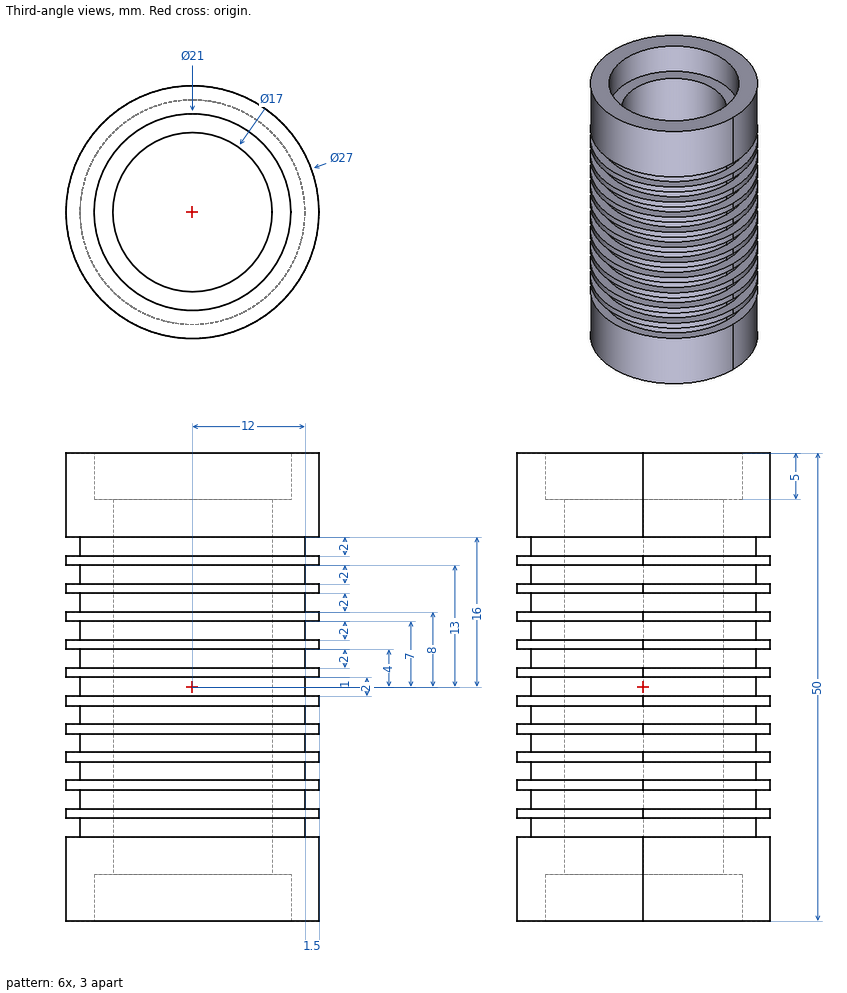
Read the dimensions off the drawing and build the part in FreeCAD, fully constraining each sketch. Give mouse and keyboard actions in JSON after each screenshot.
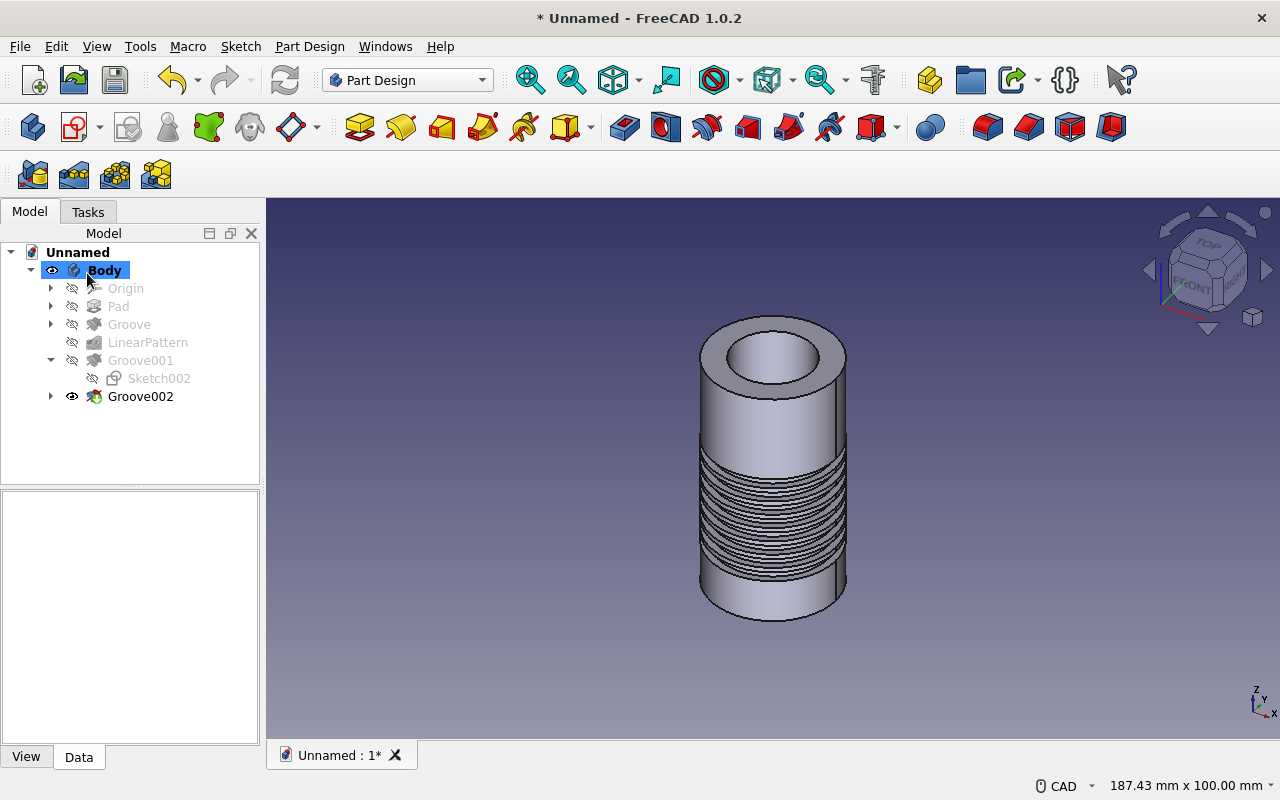
{"action": "left_click", "coordinate": [74, 128]}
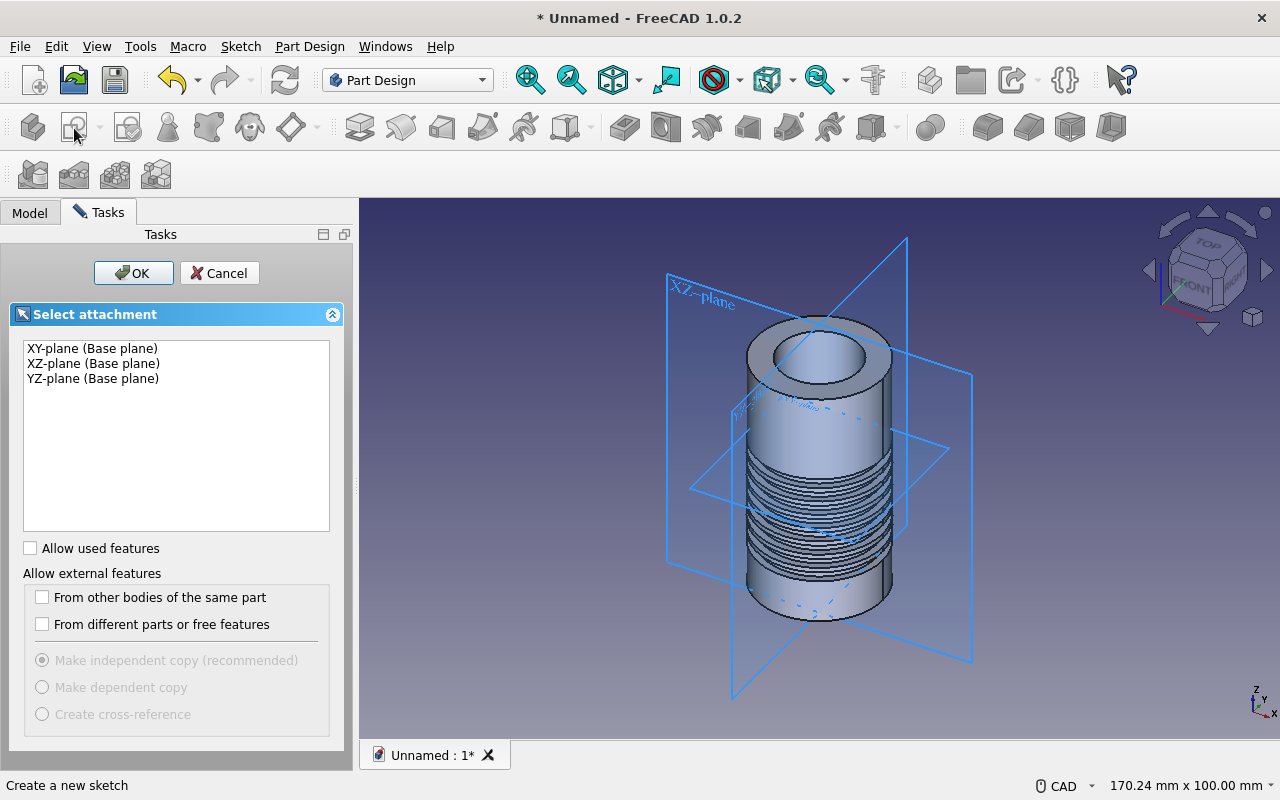
{"action": "left_click", "coordinate": [84, 364]}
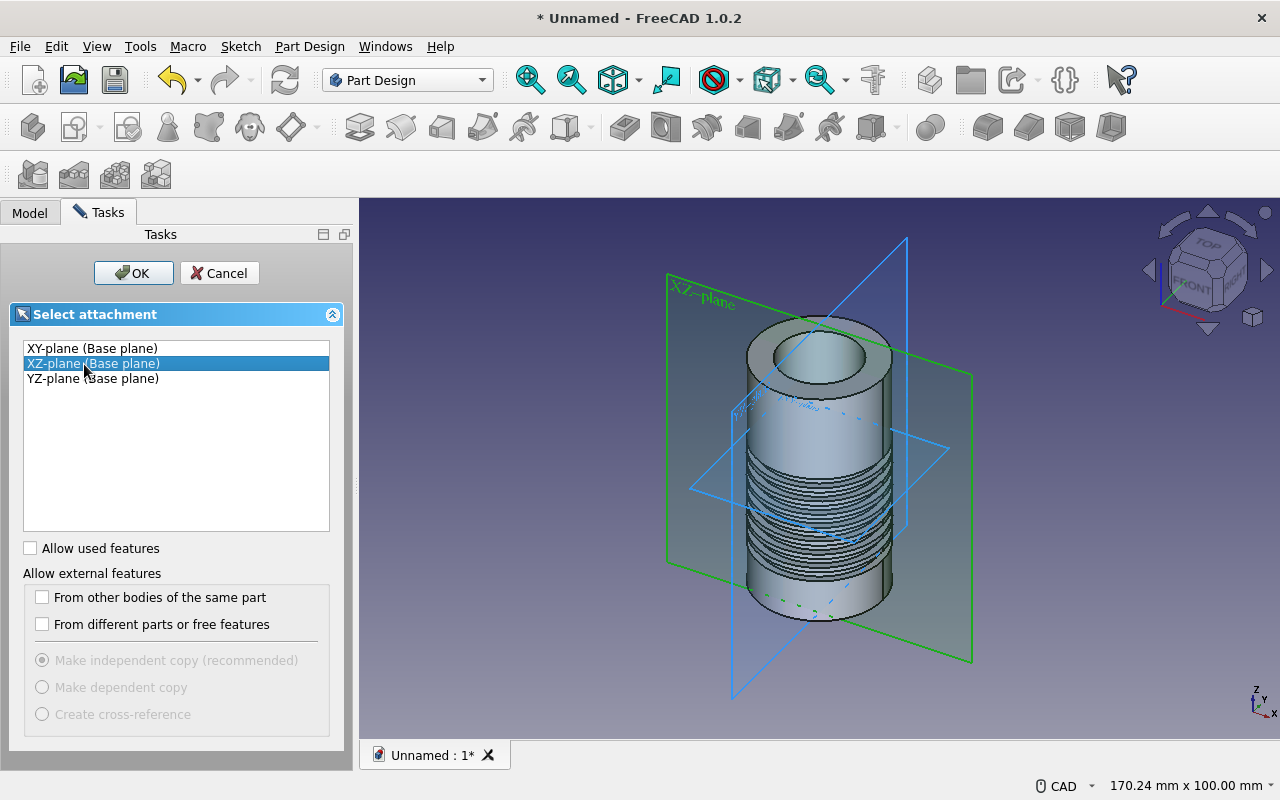
{"action": "left_click", "coordinate": [134, 273]}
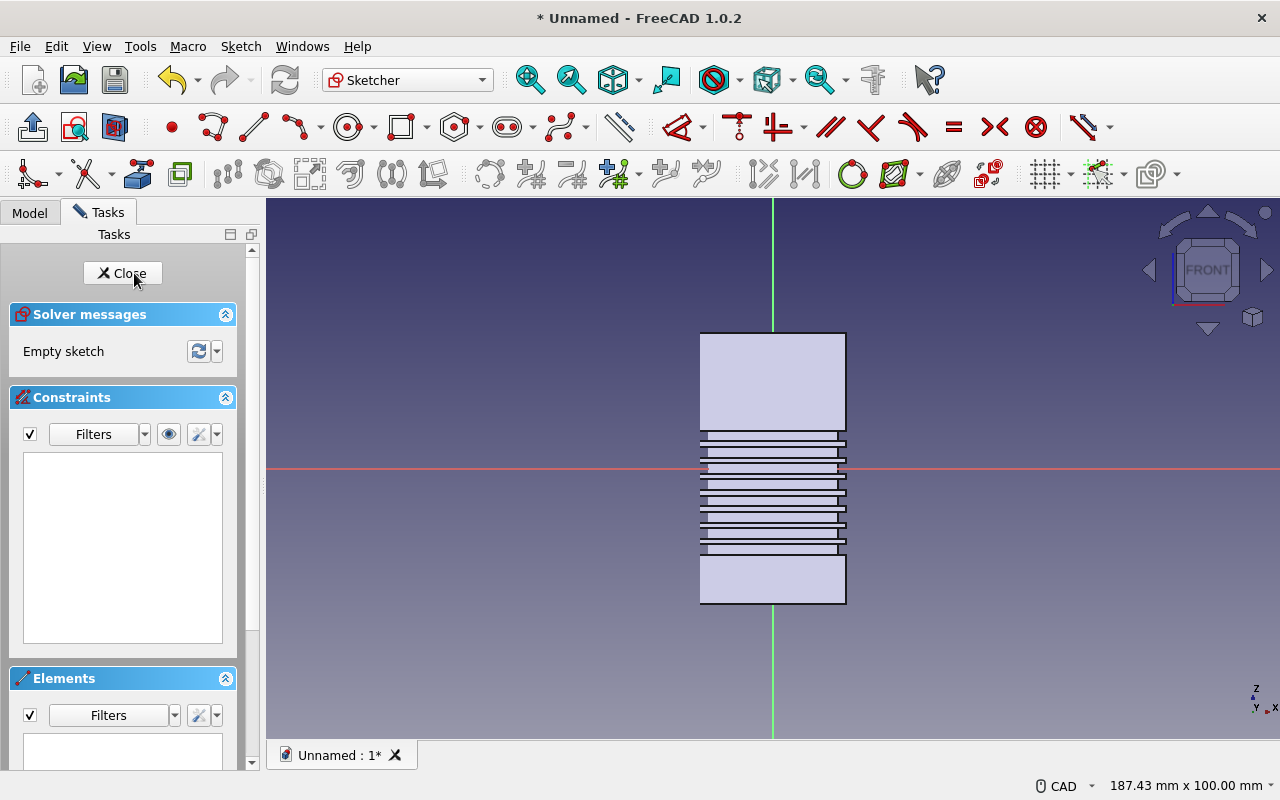
{"action": "key", "text": "q s"}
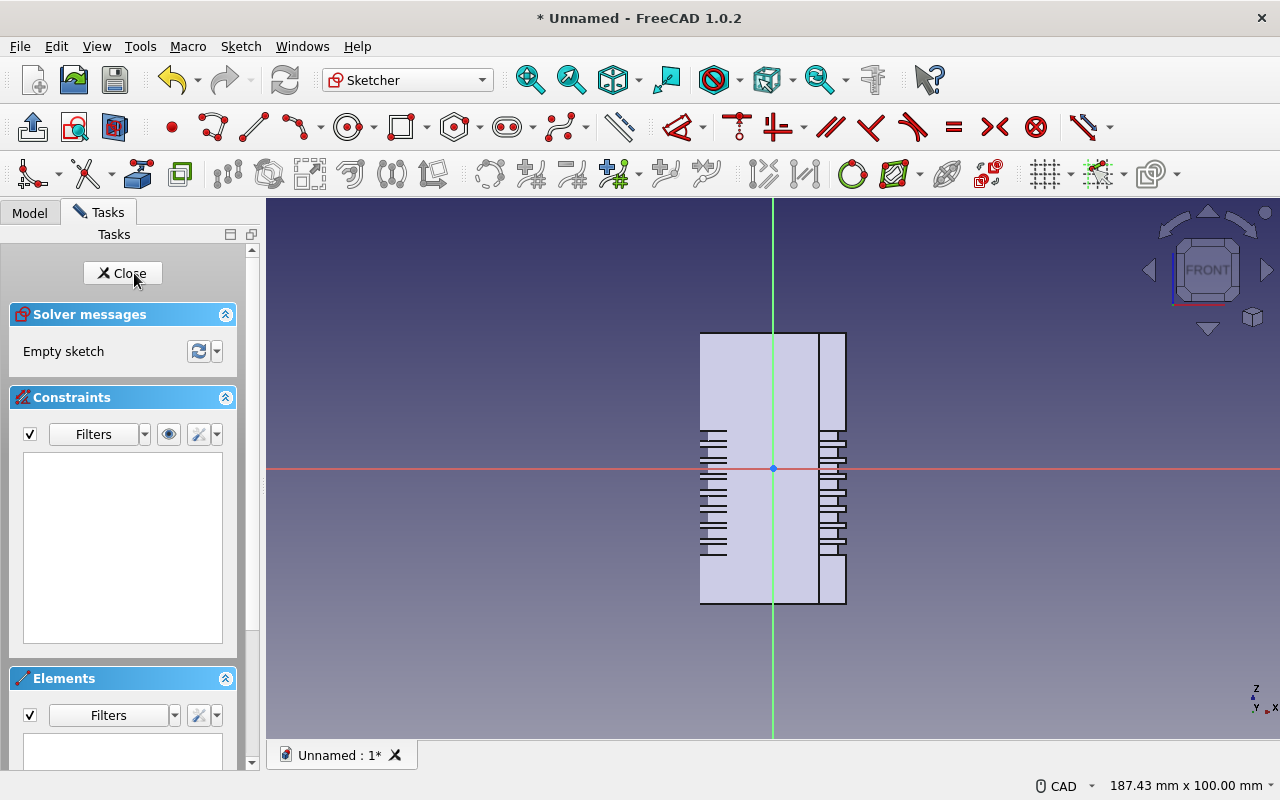
{"action": "scroll", "coordinate": [849, 417], "scroll_direction": "up", "scroll_amount": 15}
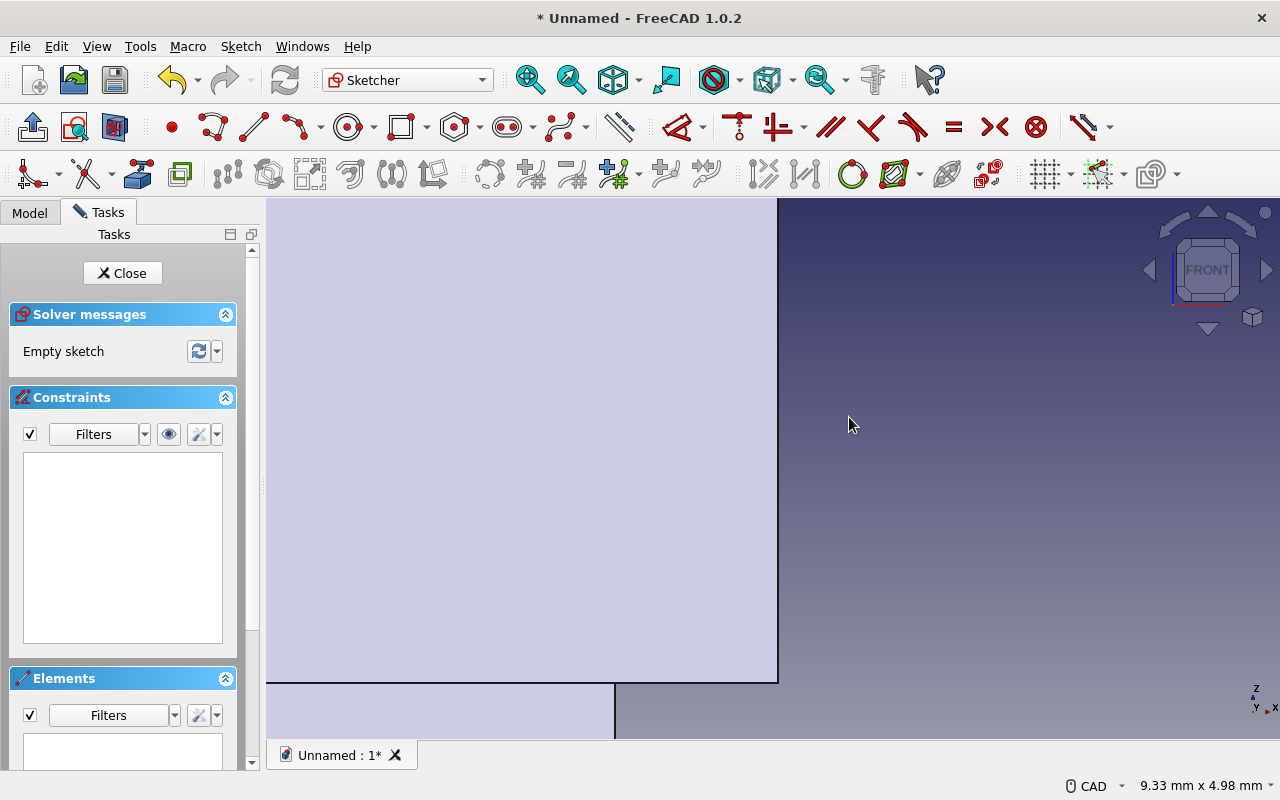
{"action": "scroll", "coordinate": [682, 460], "scroll_direction": "up", "scroll_amount": 2}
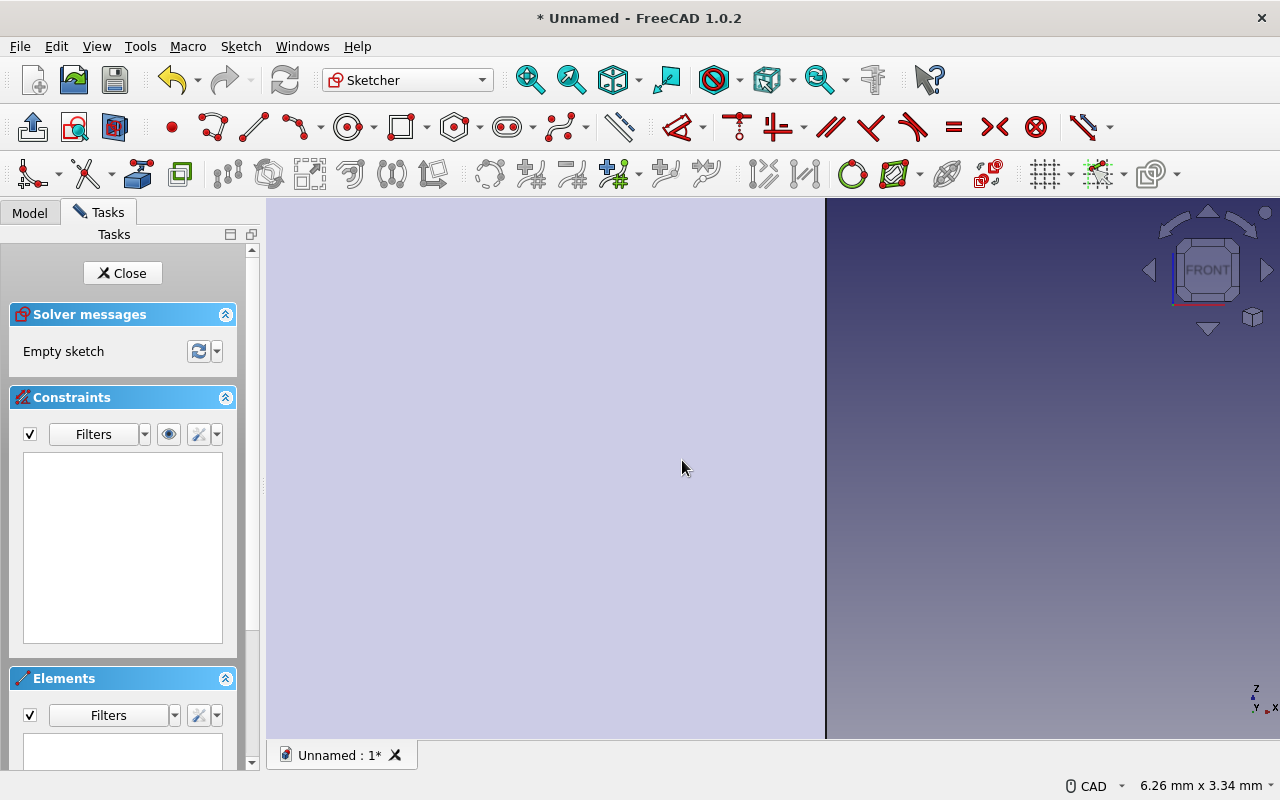
{"action": "left_click", "coordinate": [400, 128]}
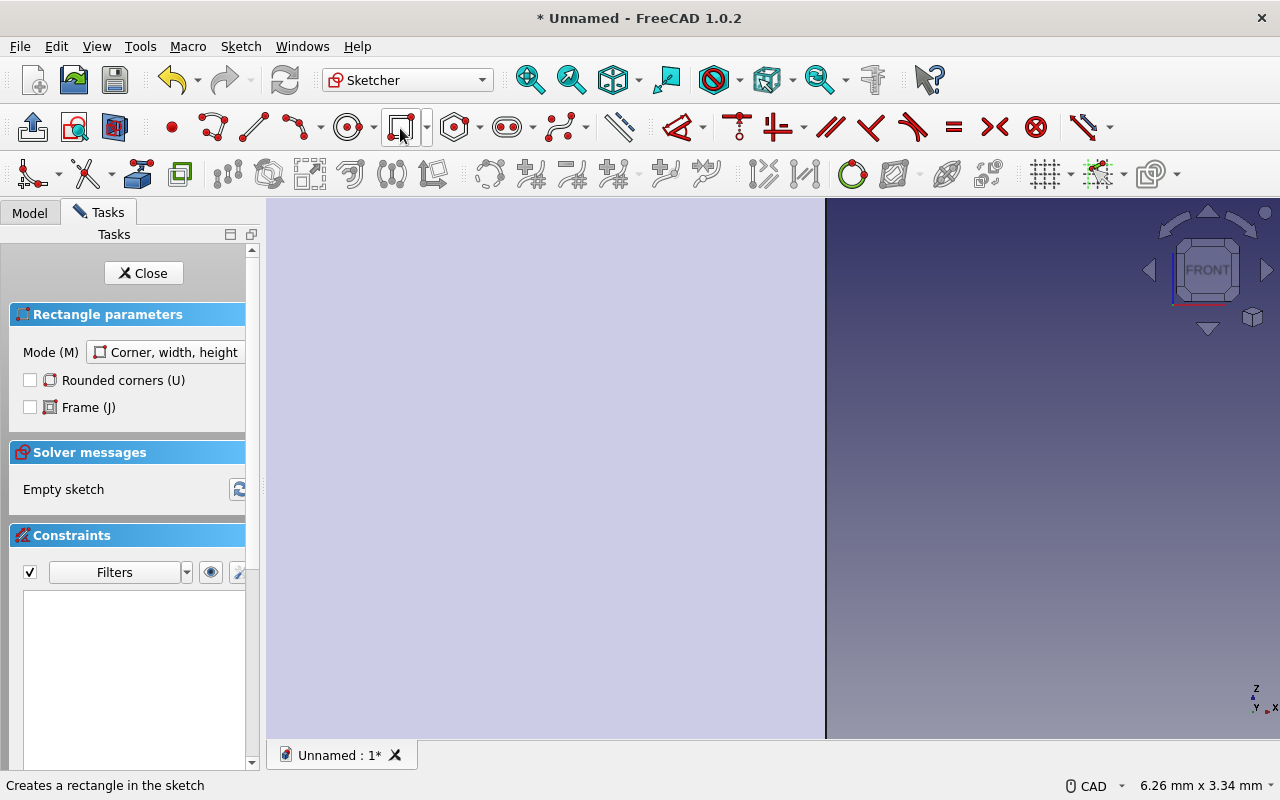
{"action": "left_click", "coordinate": [583, 306]}
{"action": "mouse_move", "coordinate": [826, 630]}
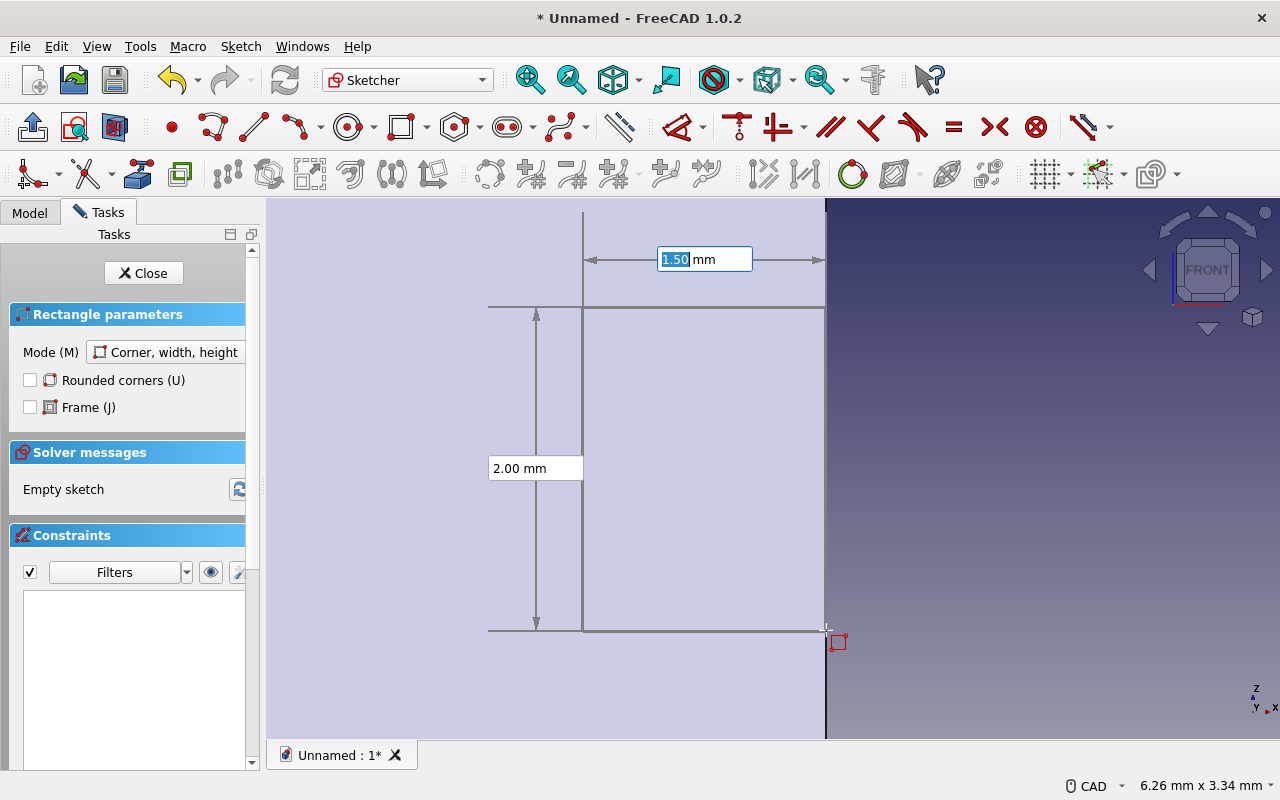
{"action": "type", "text": "1.5"}
{"action": "key", "text": "Tab"}
{"action": "type", "text": "2"}
{"action": "key", "text": "Return"}
{"action": "key", "text": "Escape"}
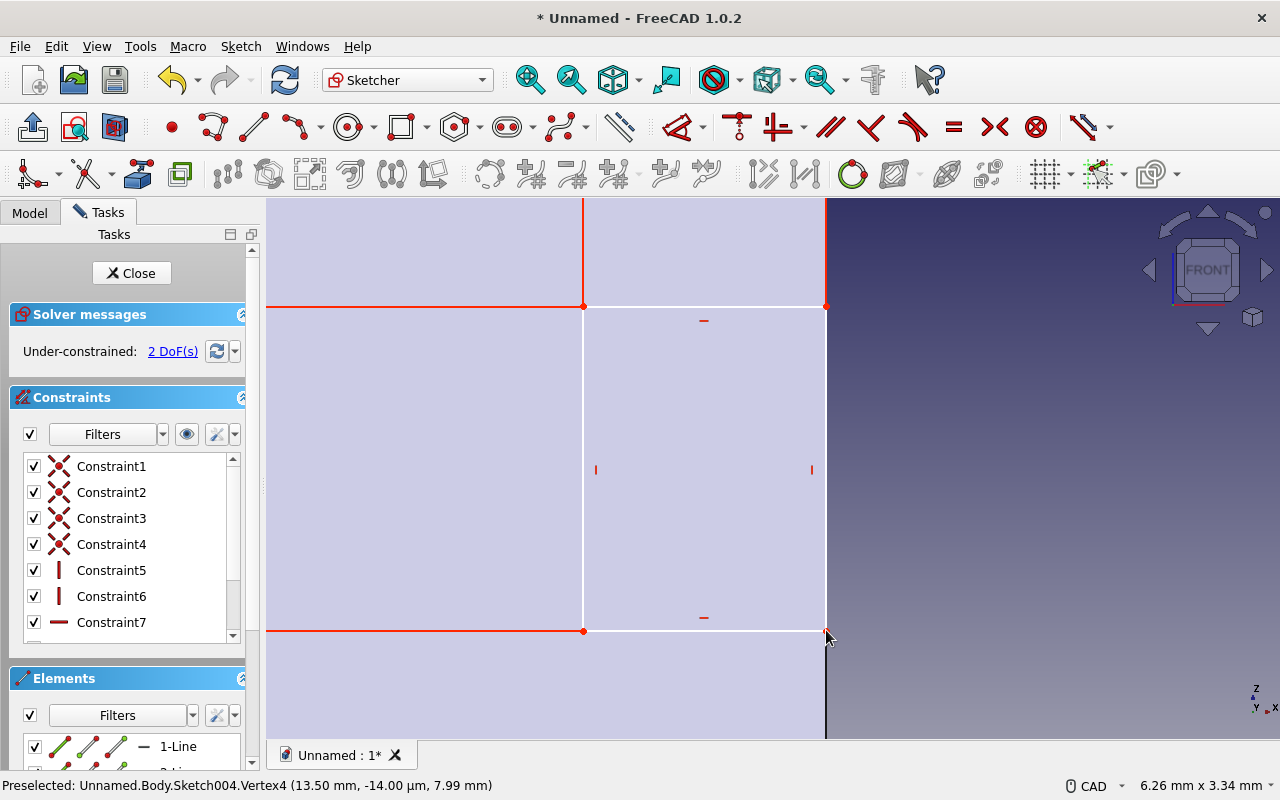
{"action": "left_click", "coordinate": [676, 128]}